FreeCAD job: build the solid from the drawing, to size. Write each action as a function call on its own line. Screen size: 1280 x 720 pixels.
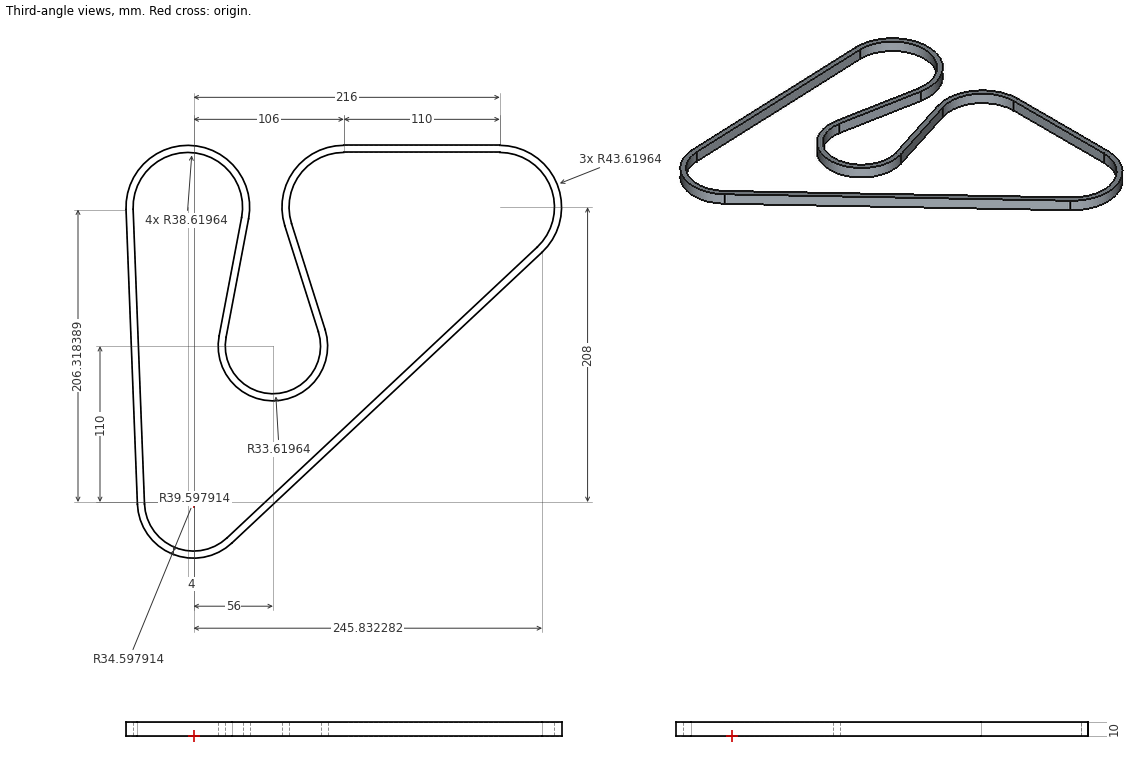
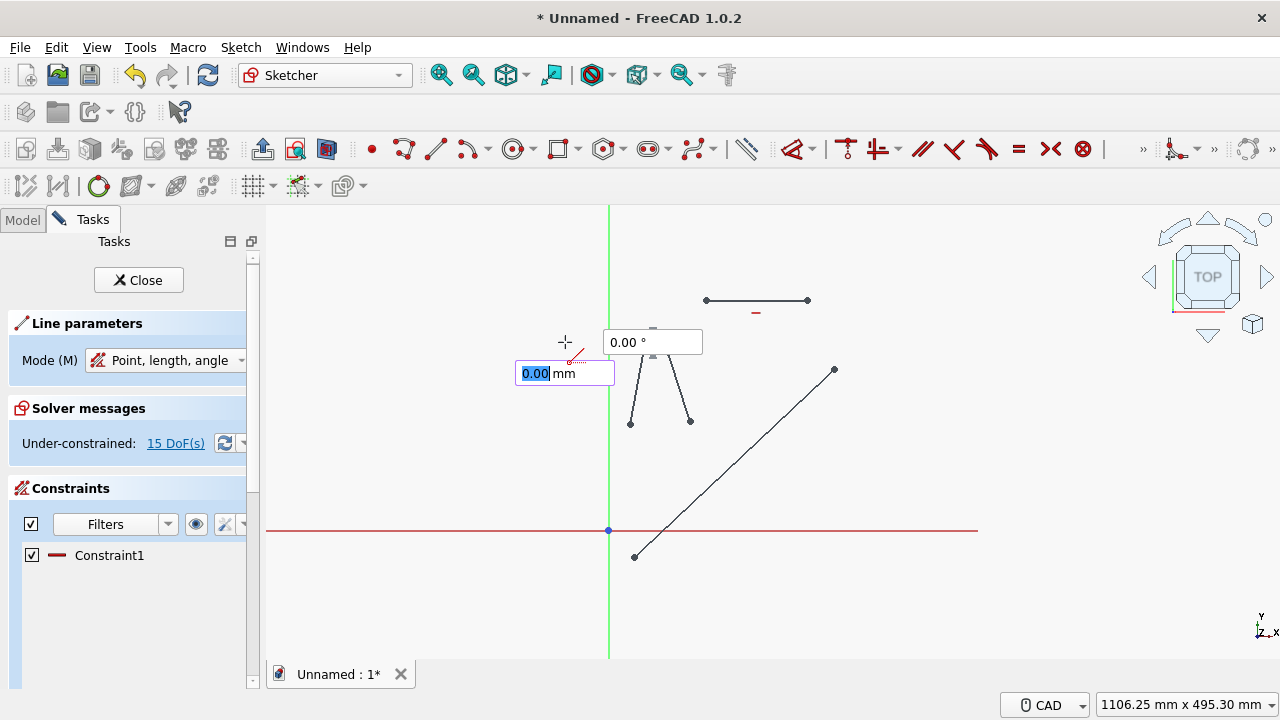
scroll(573, 532, up, 13)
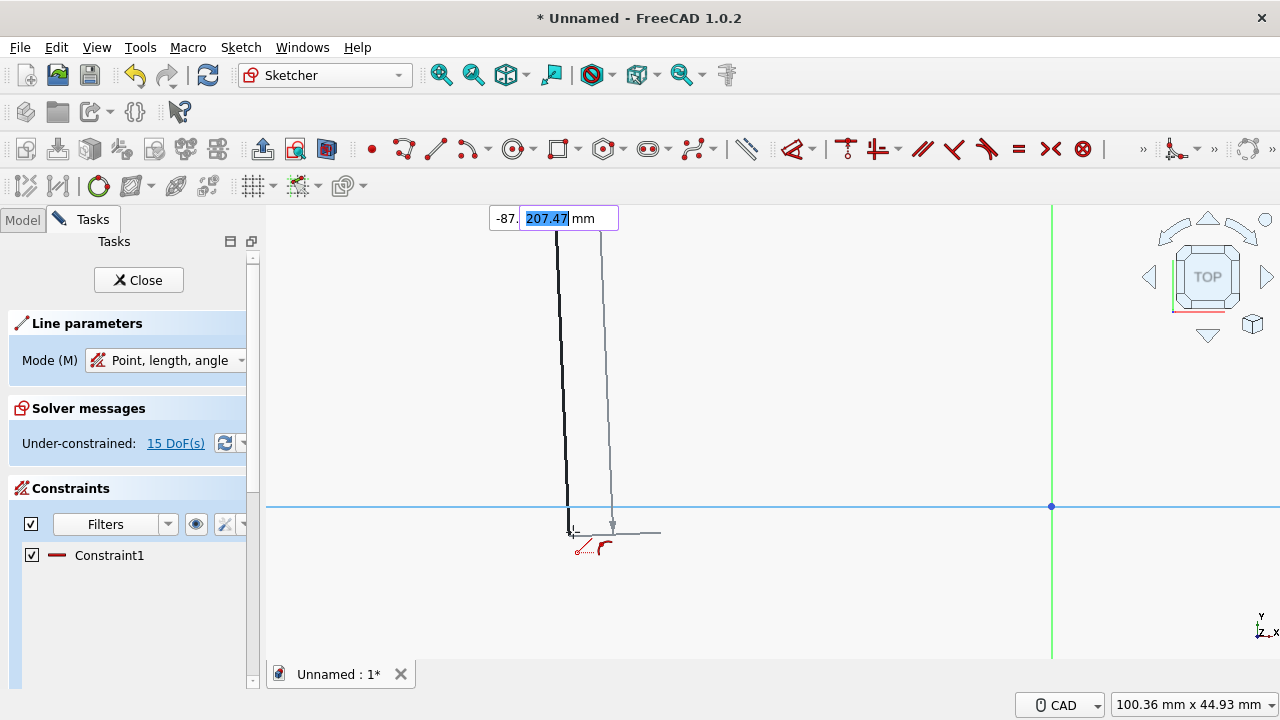
click(578, 525)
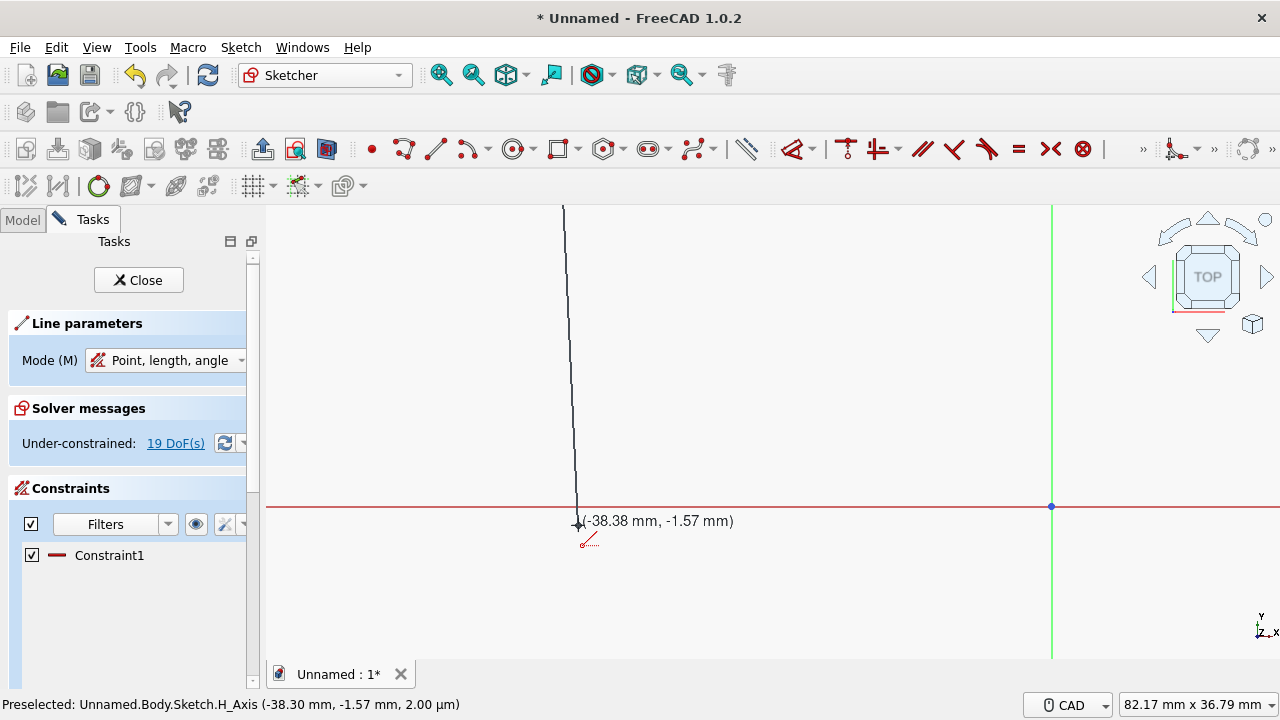
key(g)
key(3)
key(a)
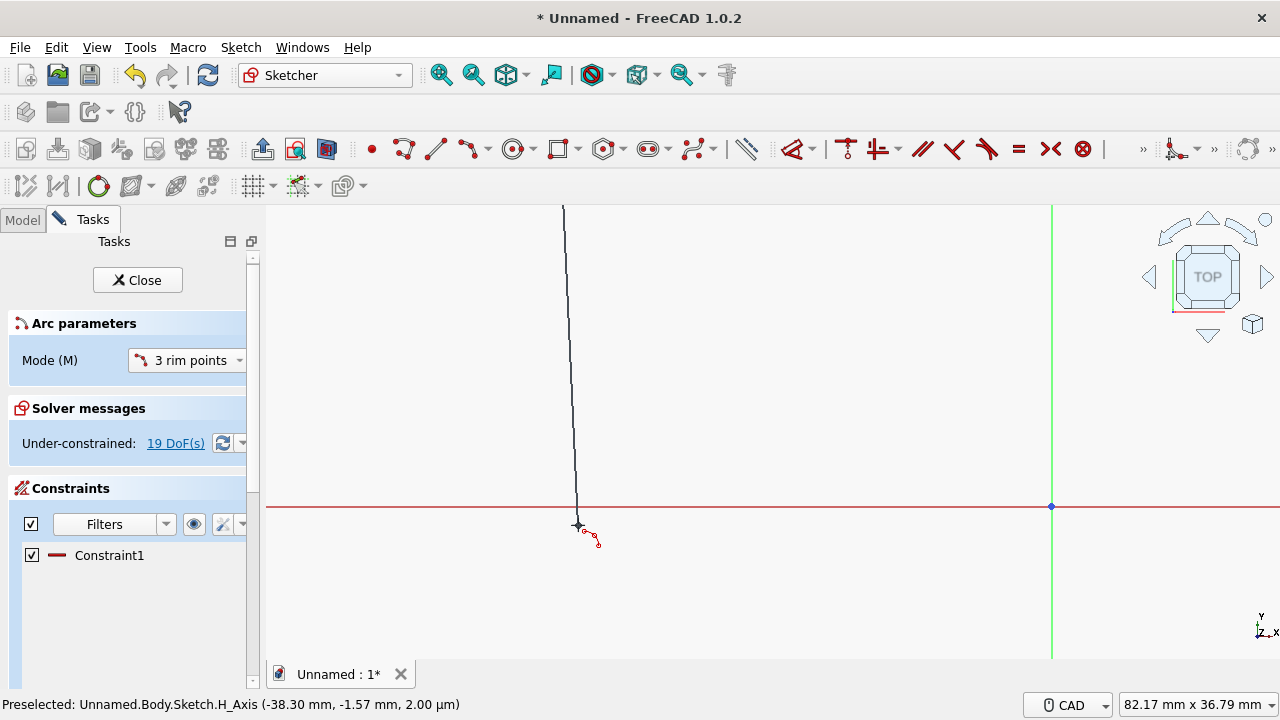
scroll(573, 532, down, 13)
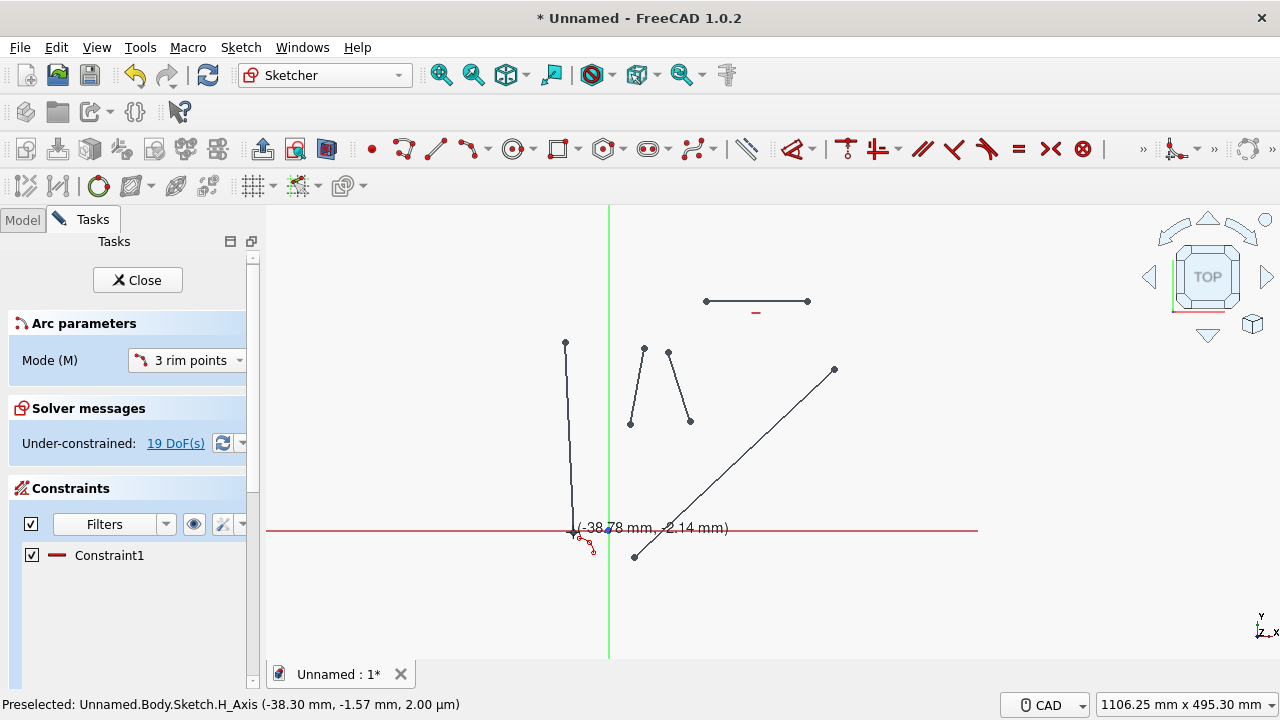
click(834, 370)
click(807, 301)
click(844, 325)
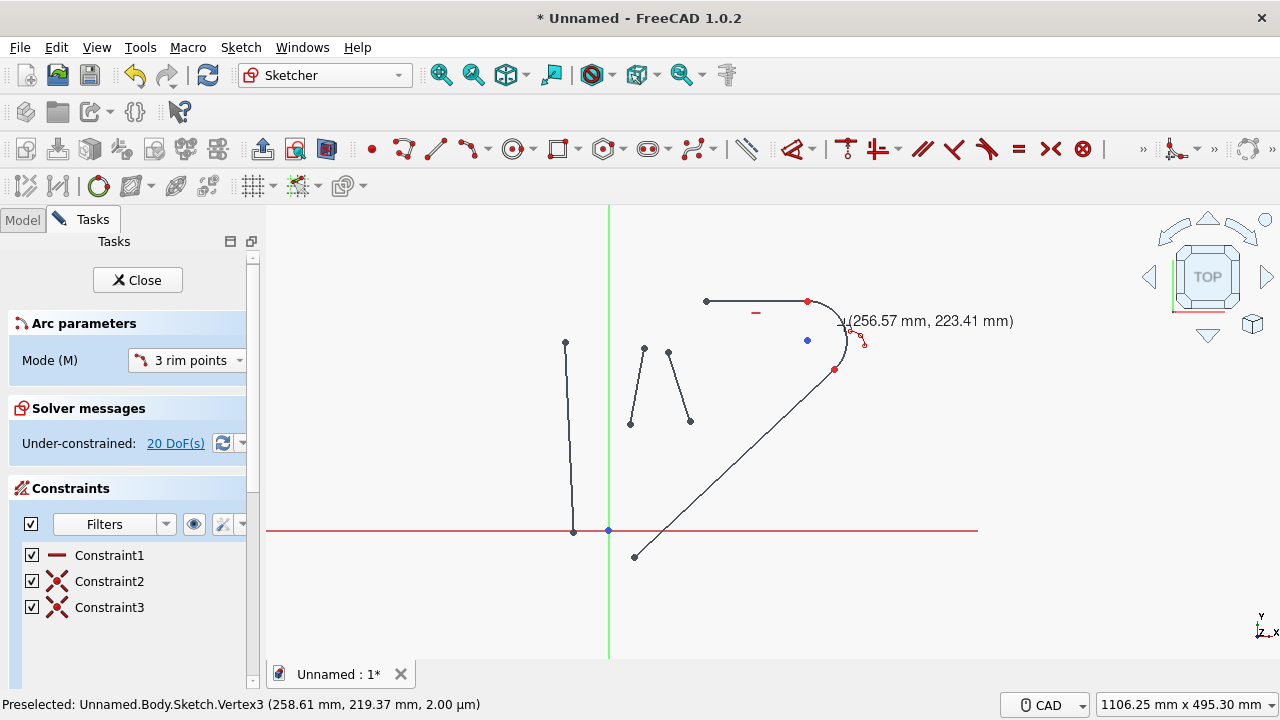
click(706, 301)
click(668, 353)
click(674, 317)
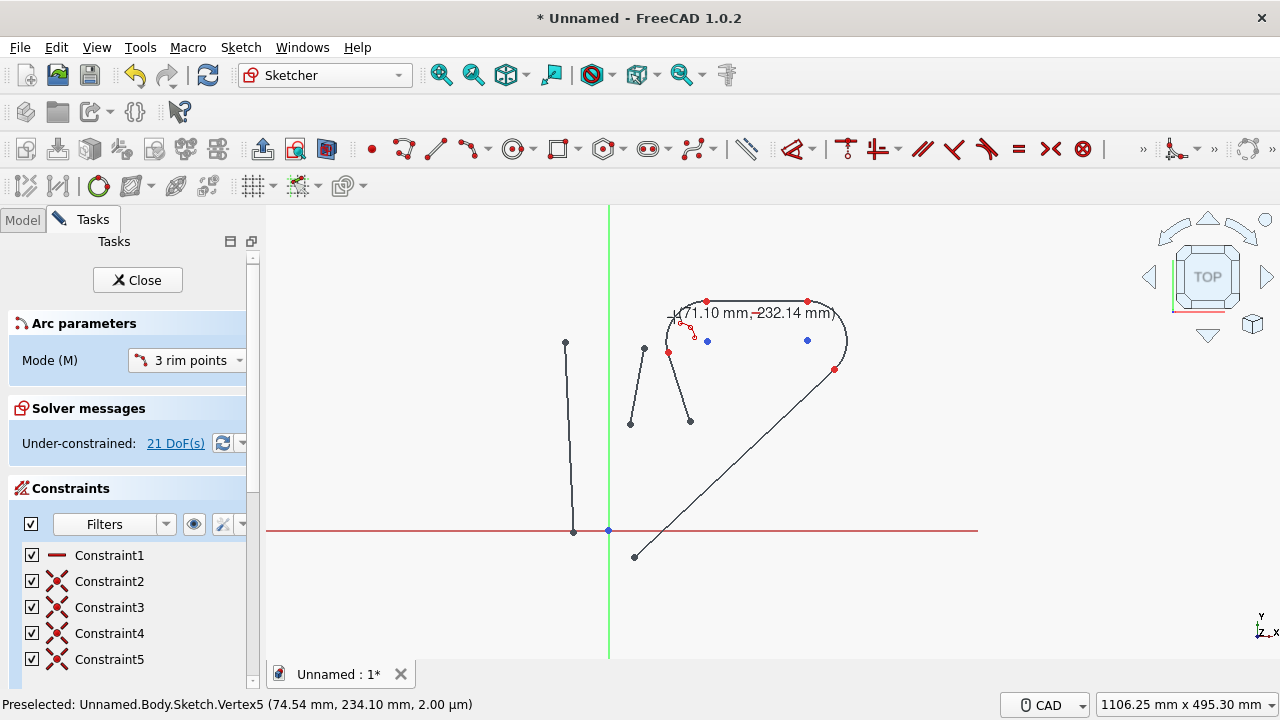
click(690, 422)
click(630, 425)
click(662, 461)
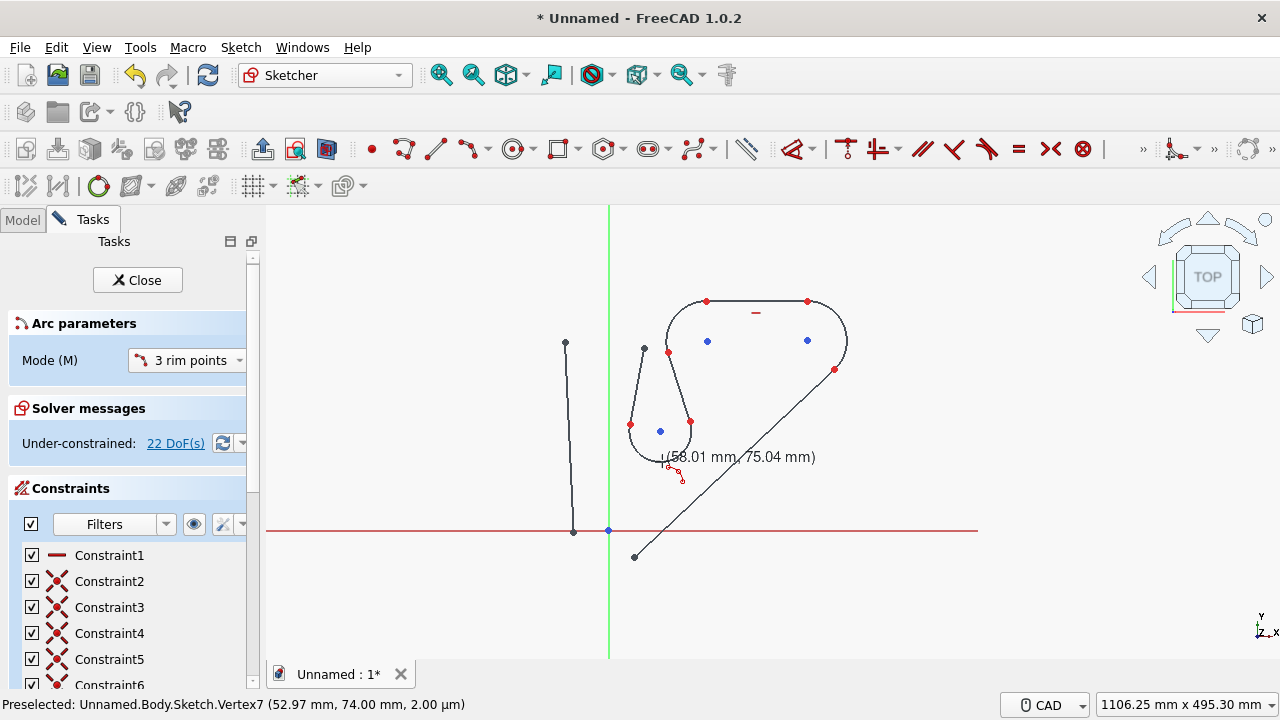
click(644, 349)
click(565, 343)
click(595, 302)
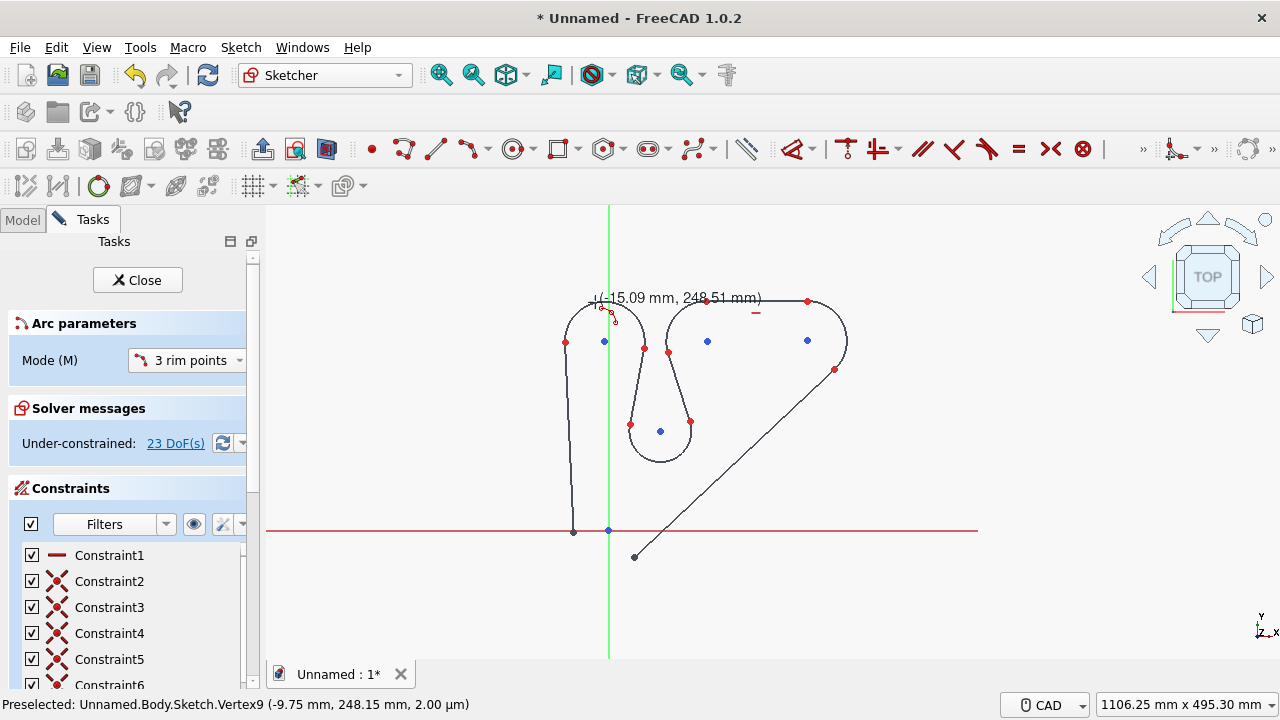
scroll(573, 532, up, 13)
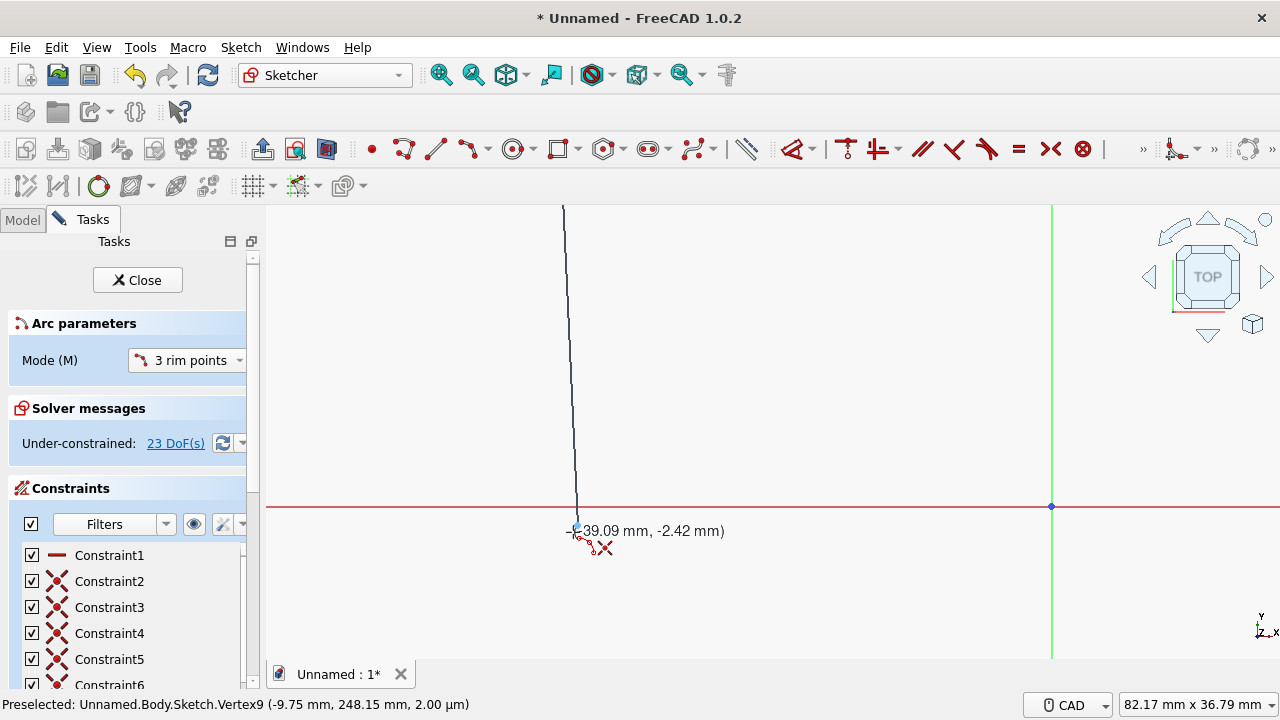
click(578, 526)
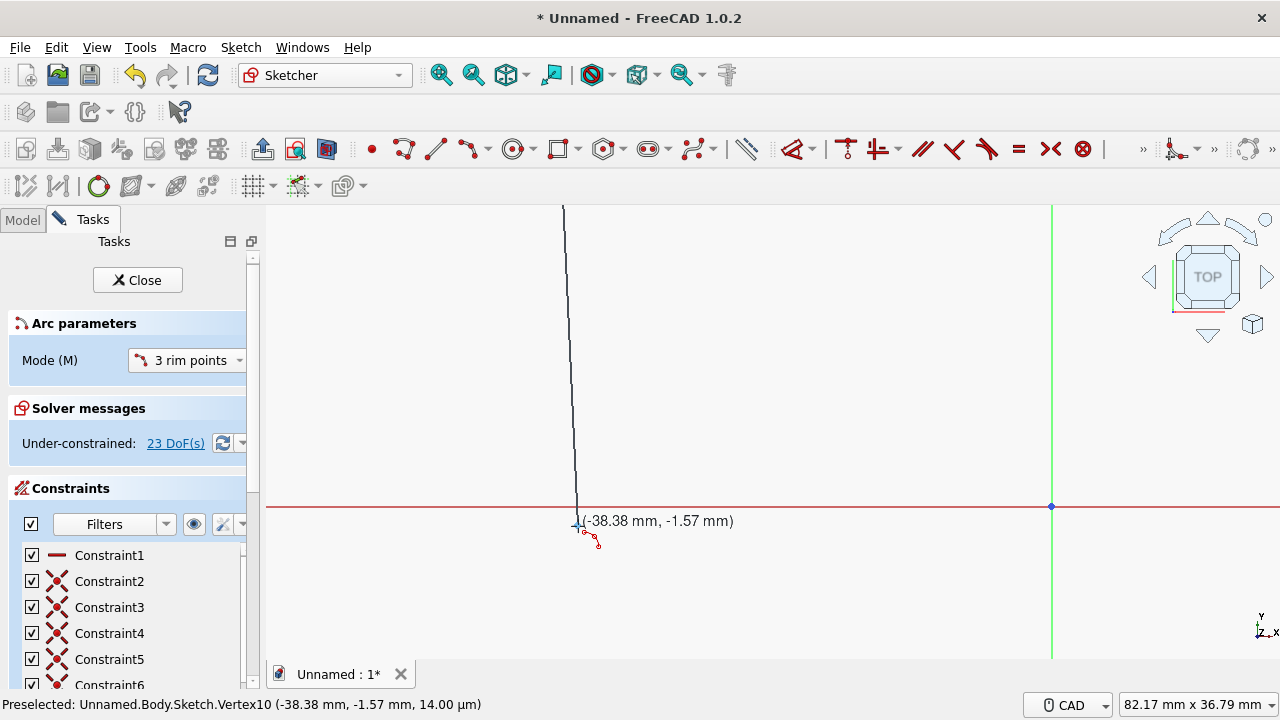
scroll(573, 532, down, 13)